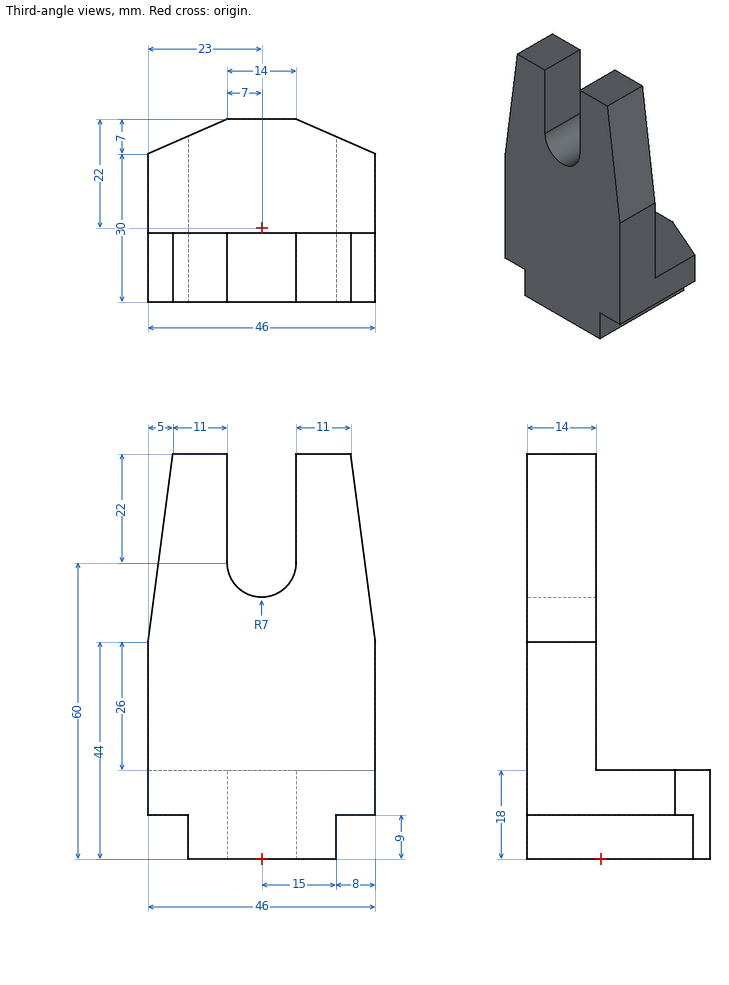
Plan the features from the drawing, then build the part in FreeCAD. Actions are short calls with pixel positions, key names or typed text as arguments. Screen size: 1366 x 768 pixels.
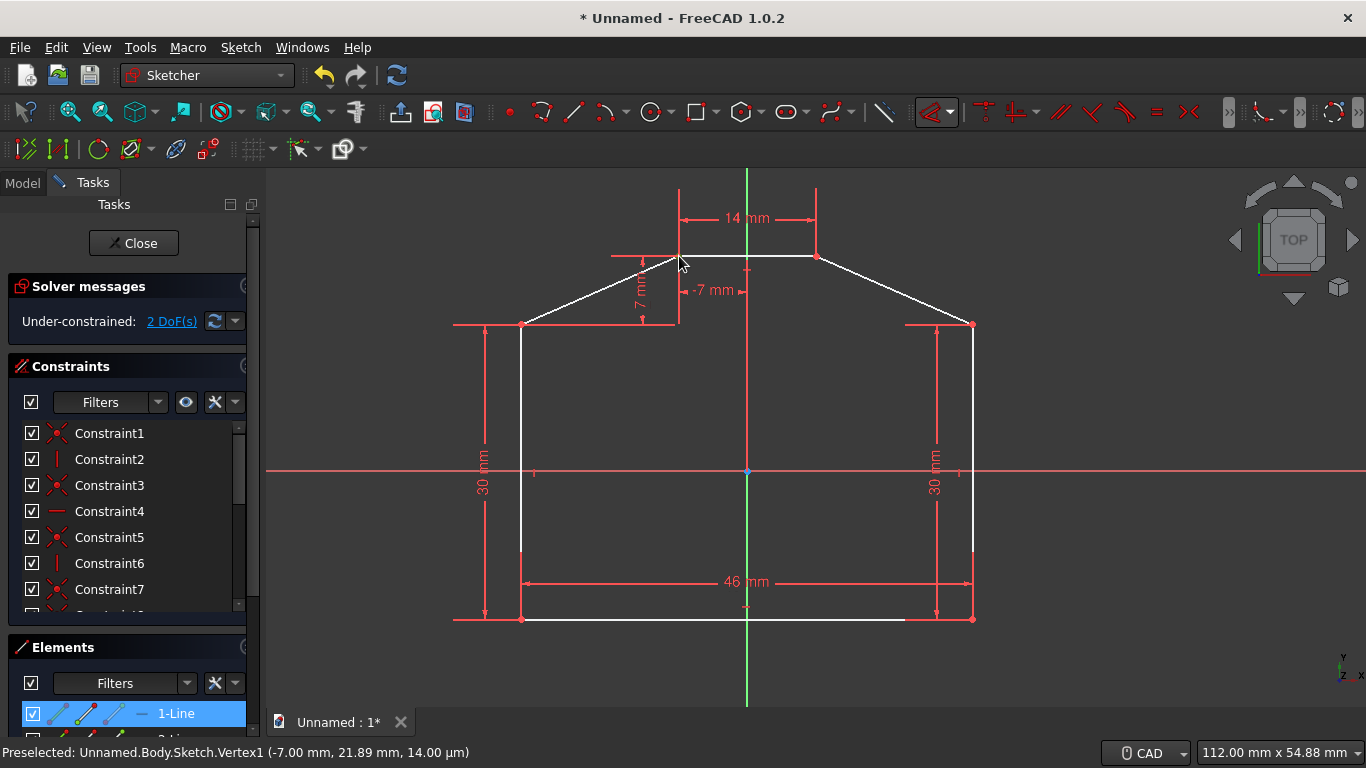
click(952, 112)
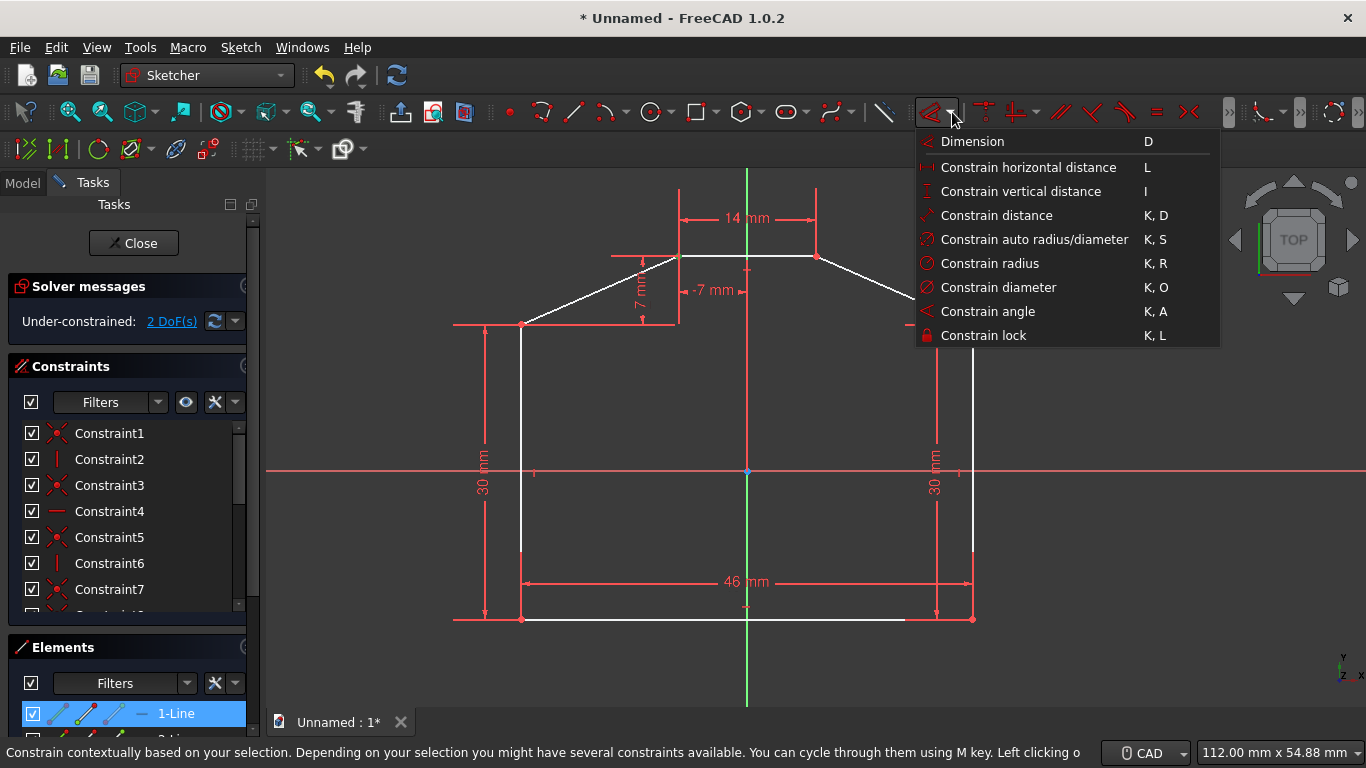
click(1068, 191)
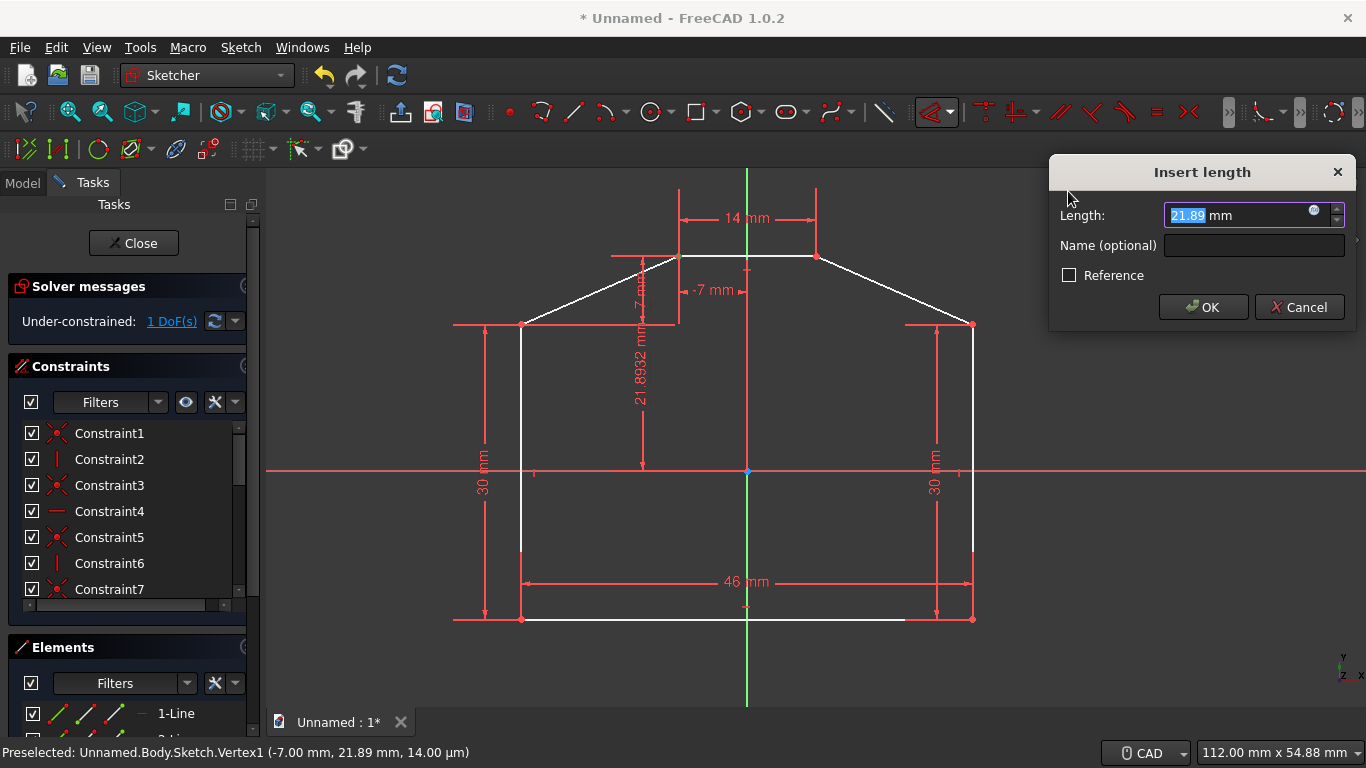
text(22)
key(Return)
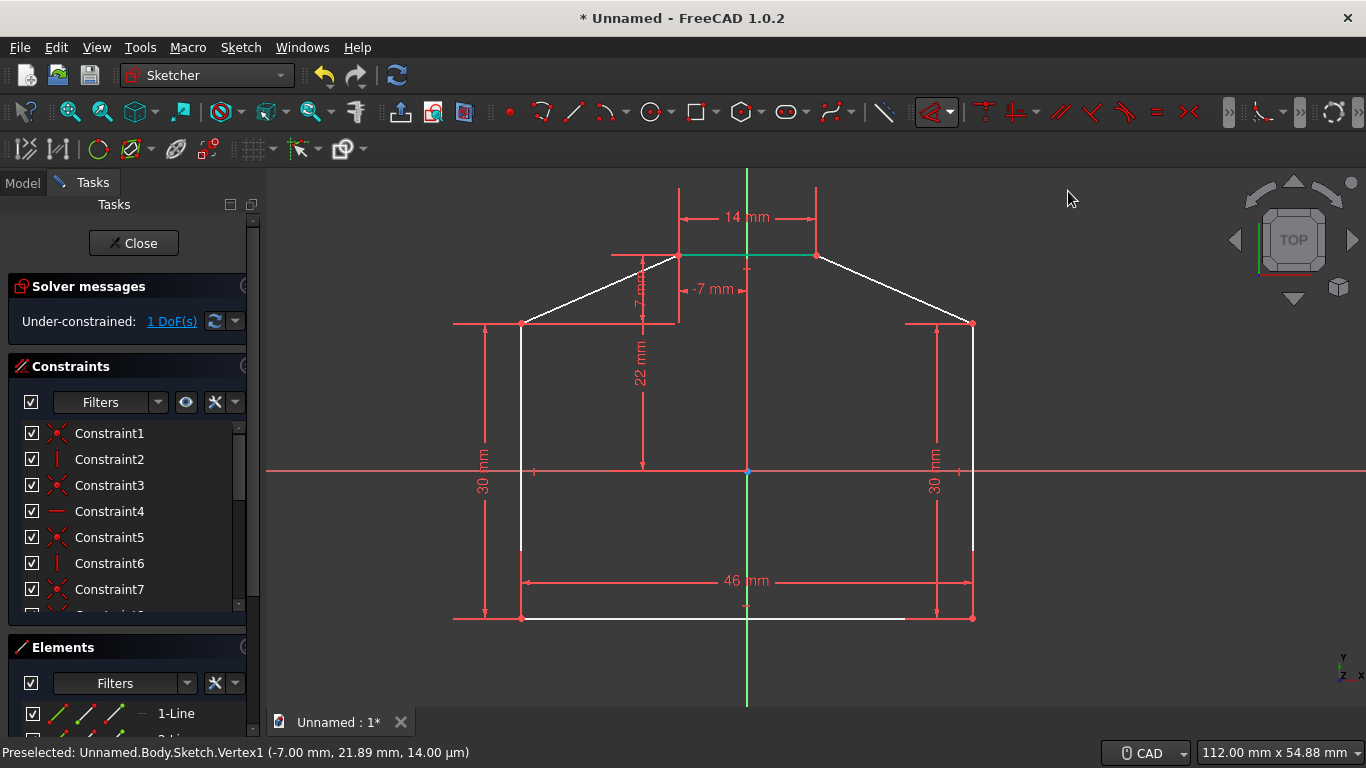
click(521, 324)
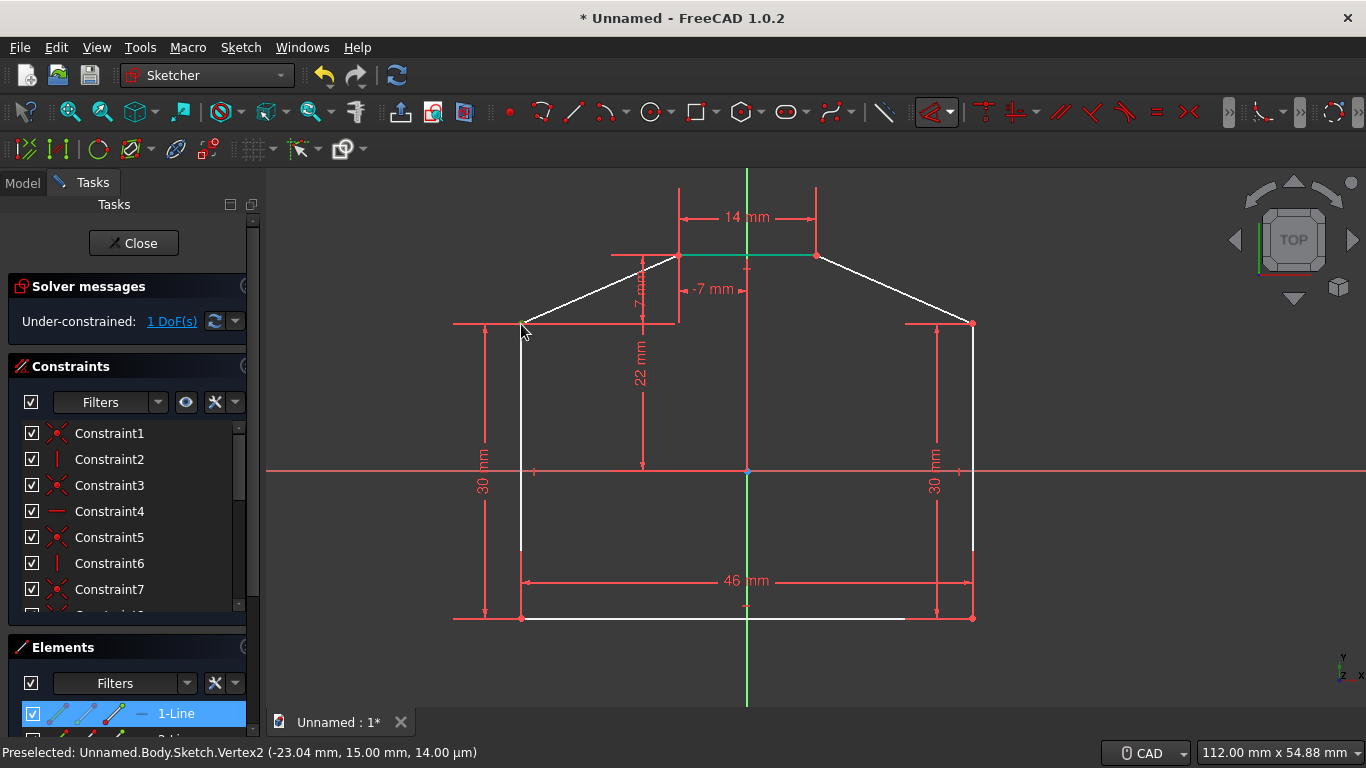
click(952, 112)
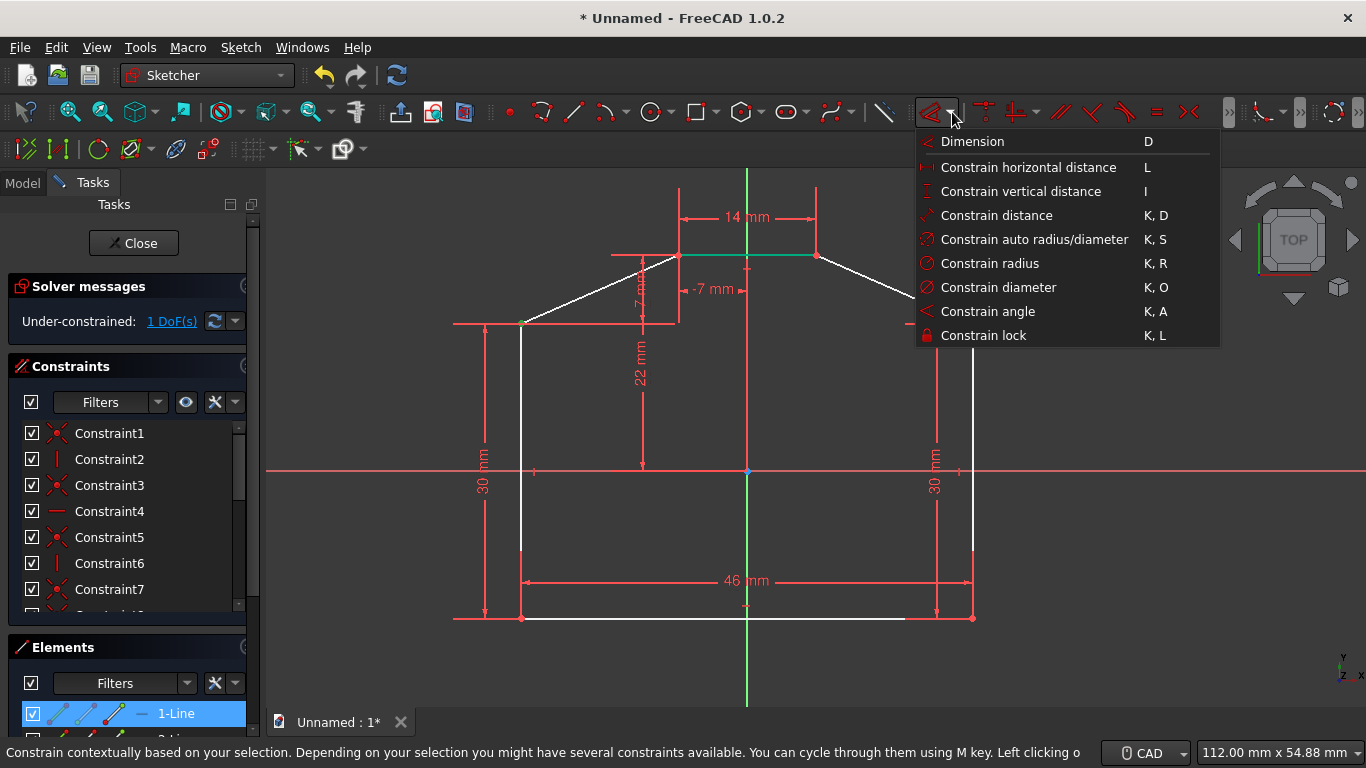
click(1068, 167)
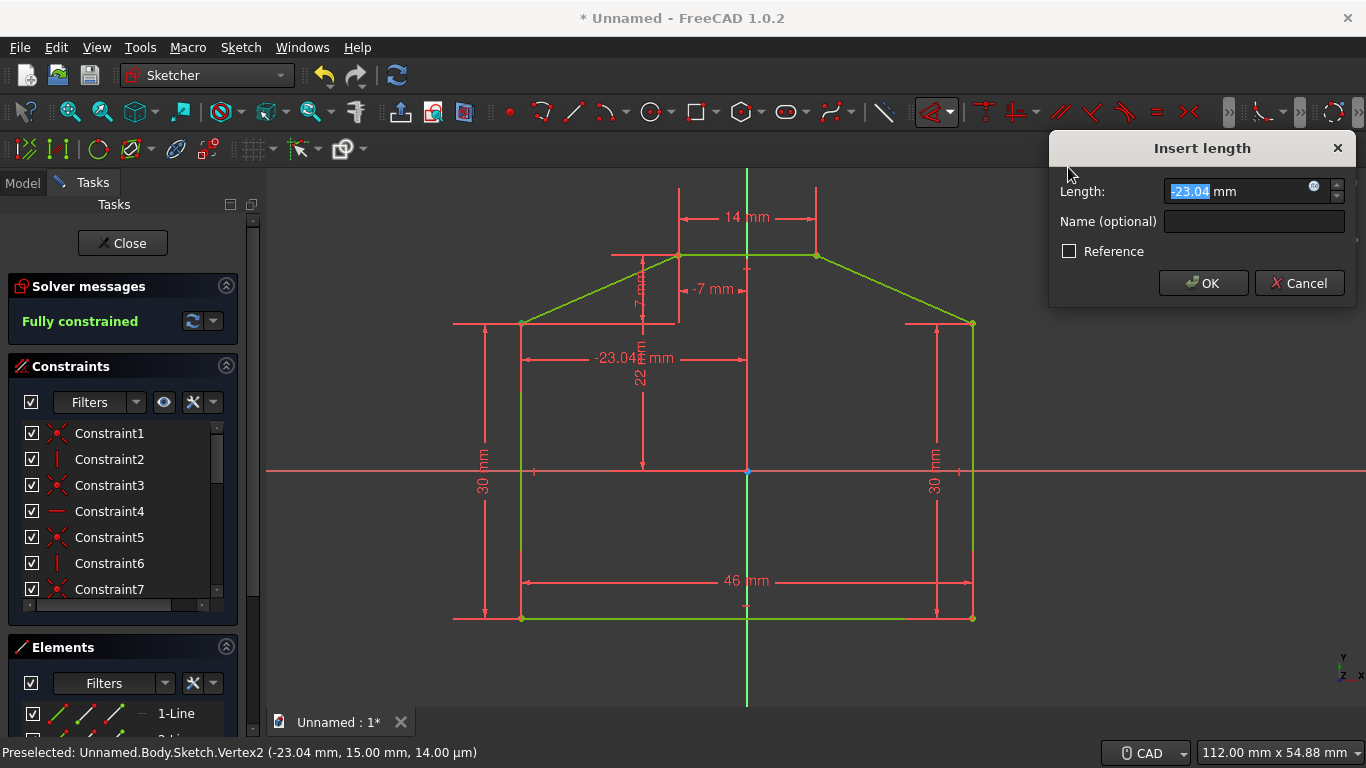
text(-23)
key(Return)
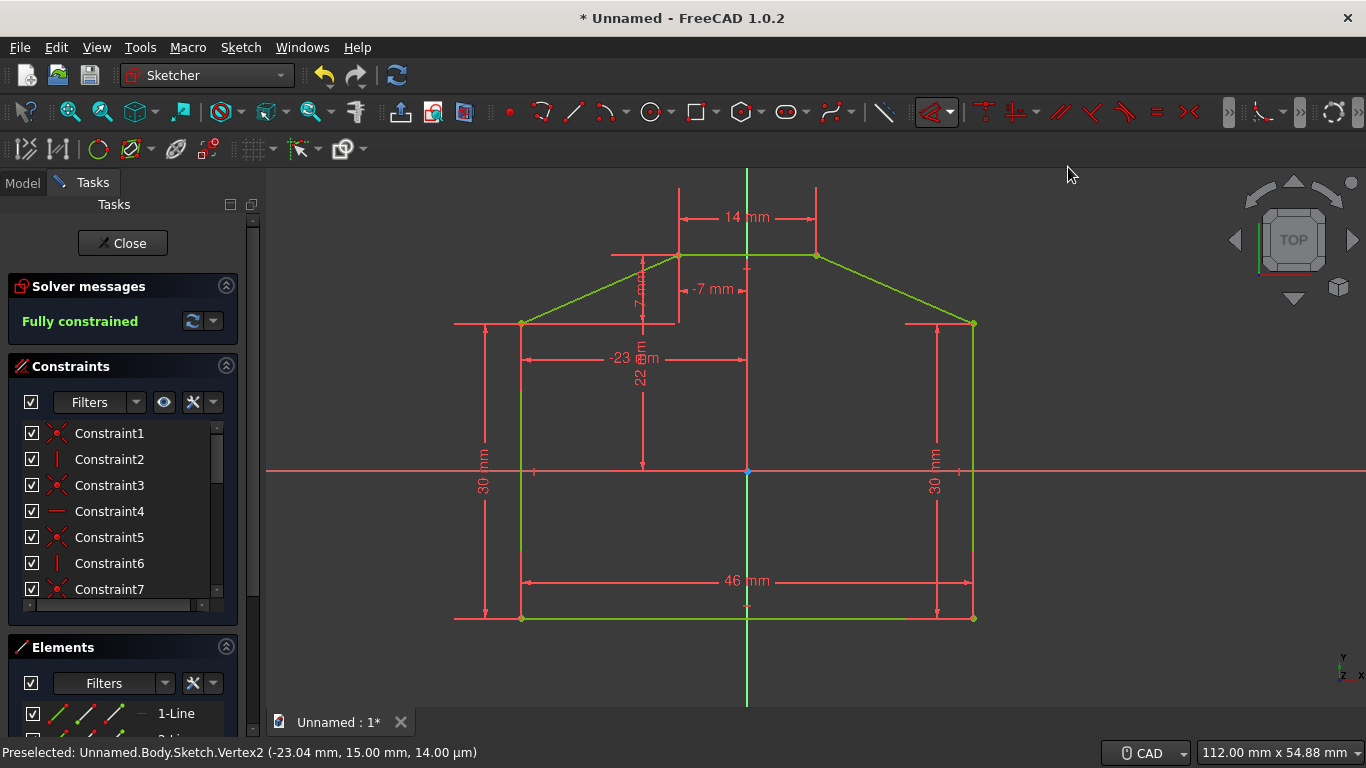
click(123, 243)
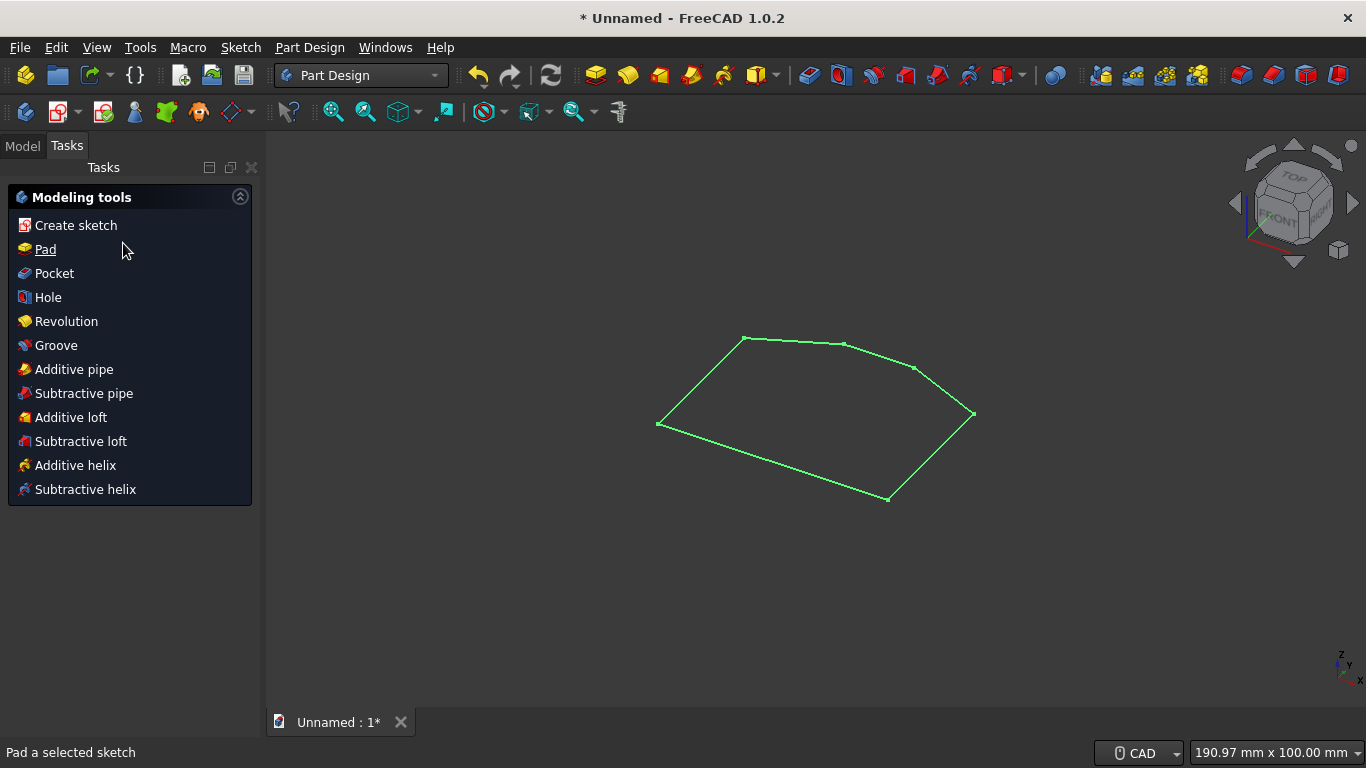
click(596, 76)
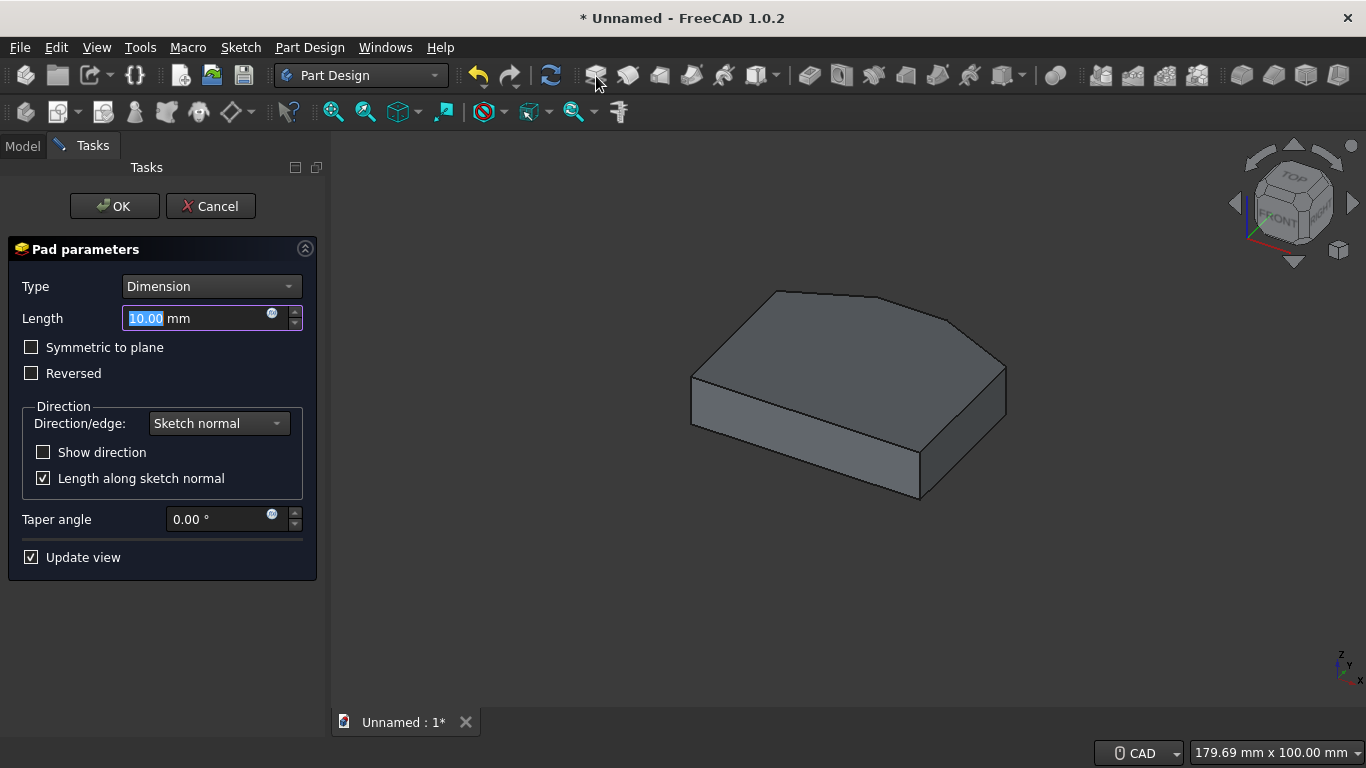
text(18)
key(Tab)